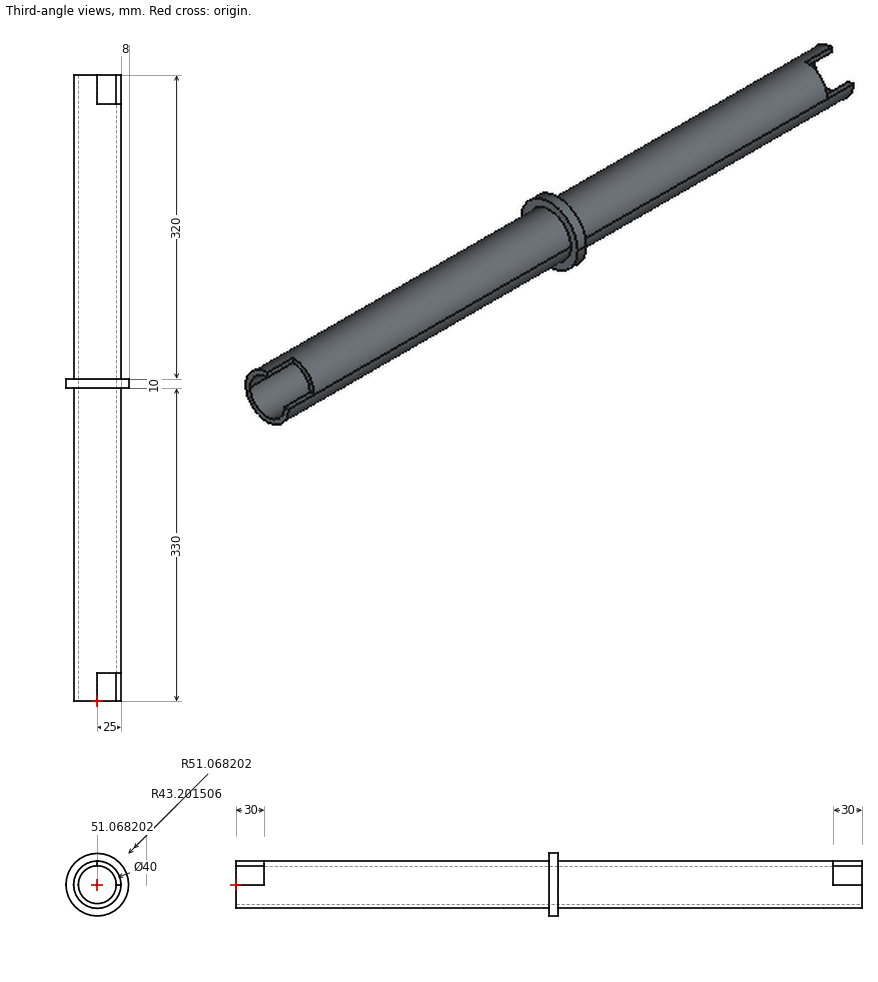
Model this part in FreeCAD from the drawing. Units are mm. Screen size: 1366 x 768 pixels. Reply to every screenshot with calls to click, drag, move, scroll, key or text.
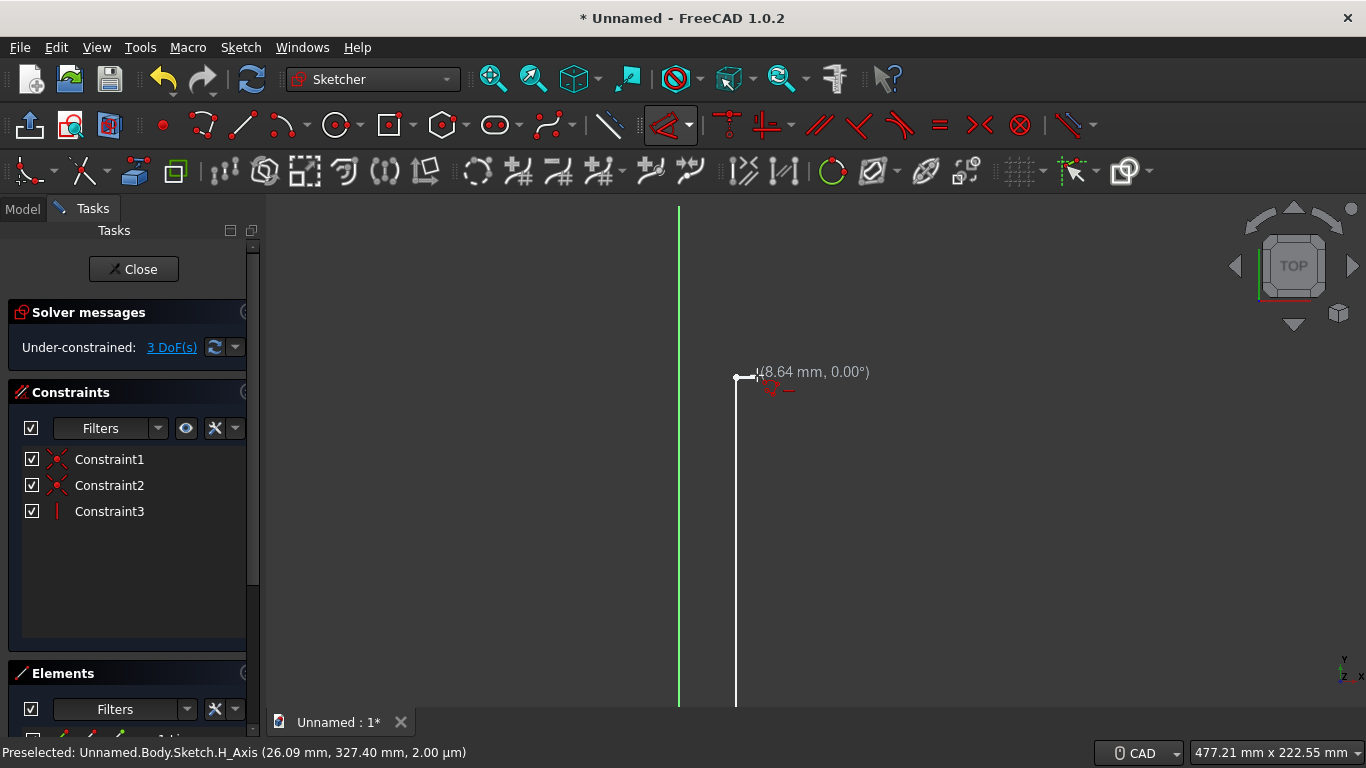
click(755, 374)
click(755, 352)
click(737, 352)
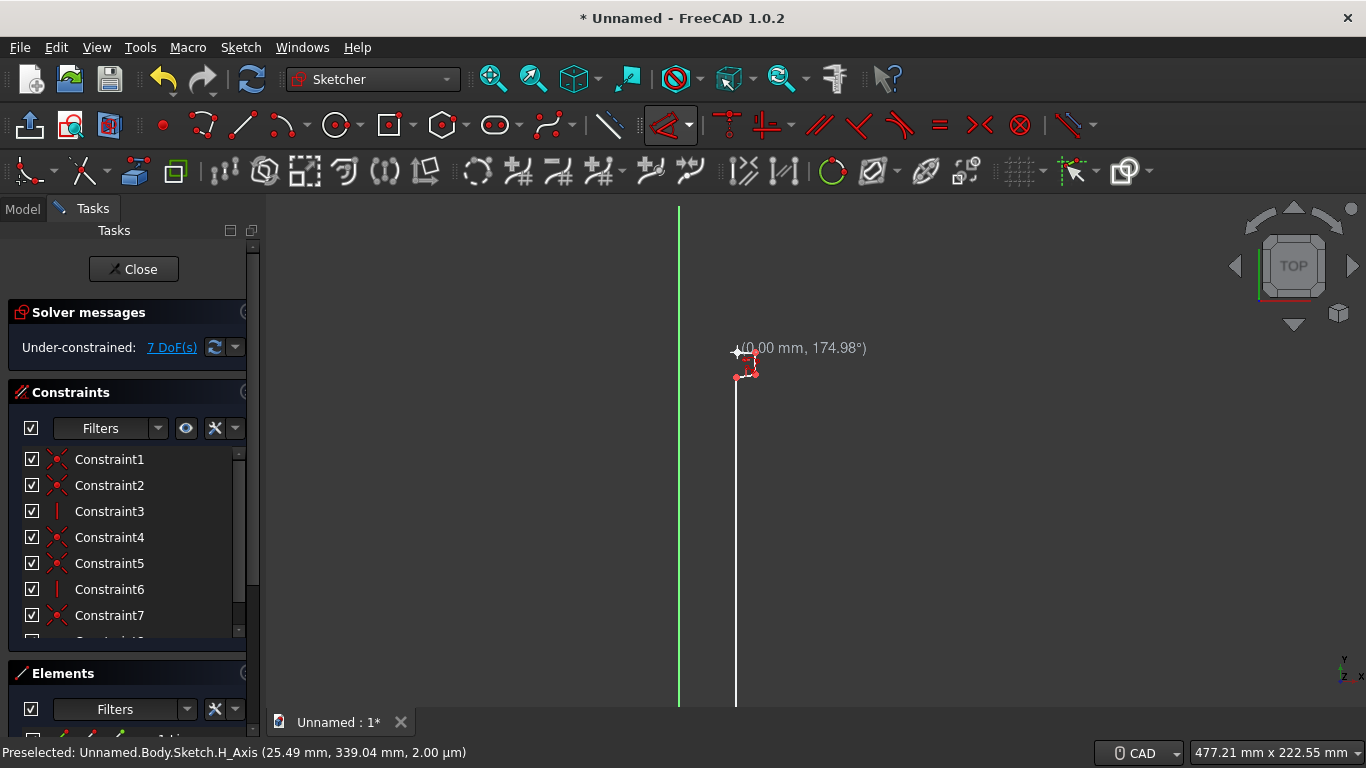
scroll(755, 470, down, 8)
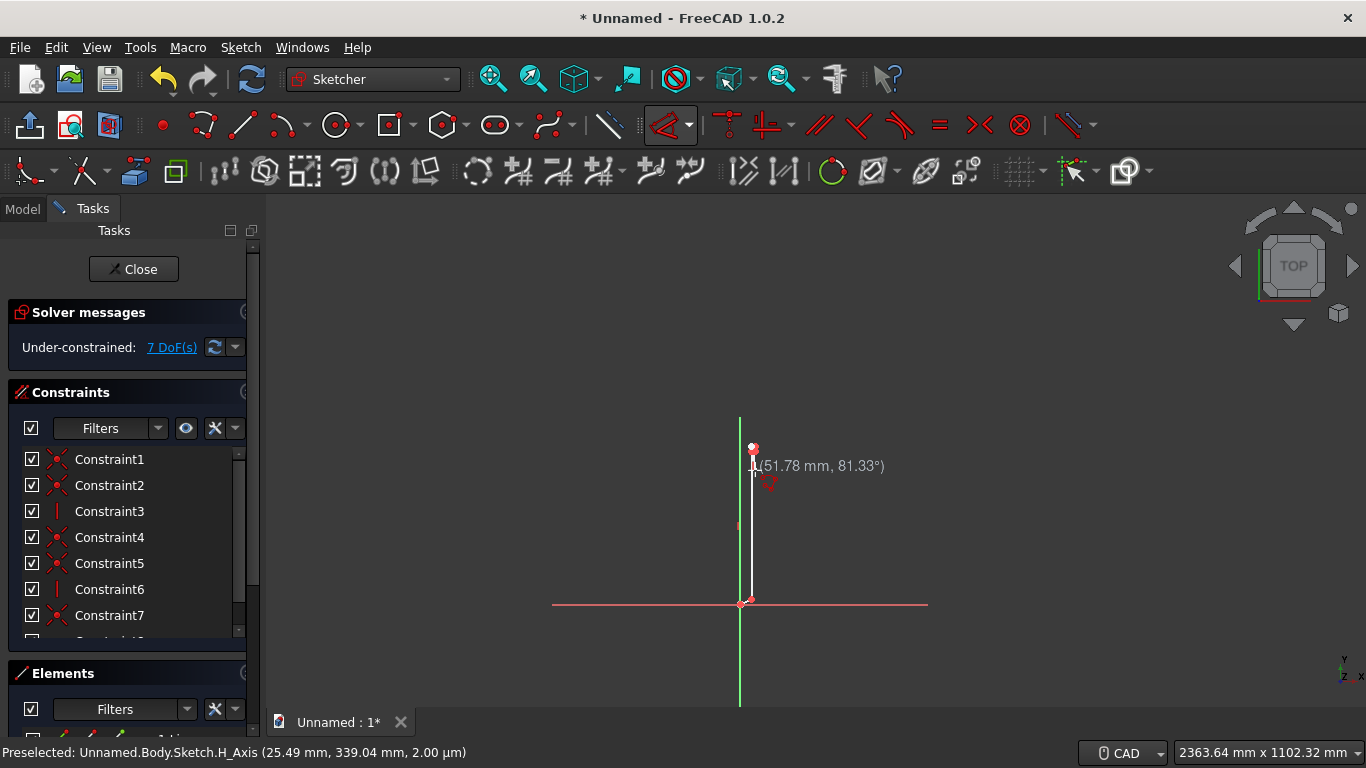
scroll(752, 298, up, 2)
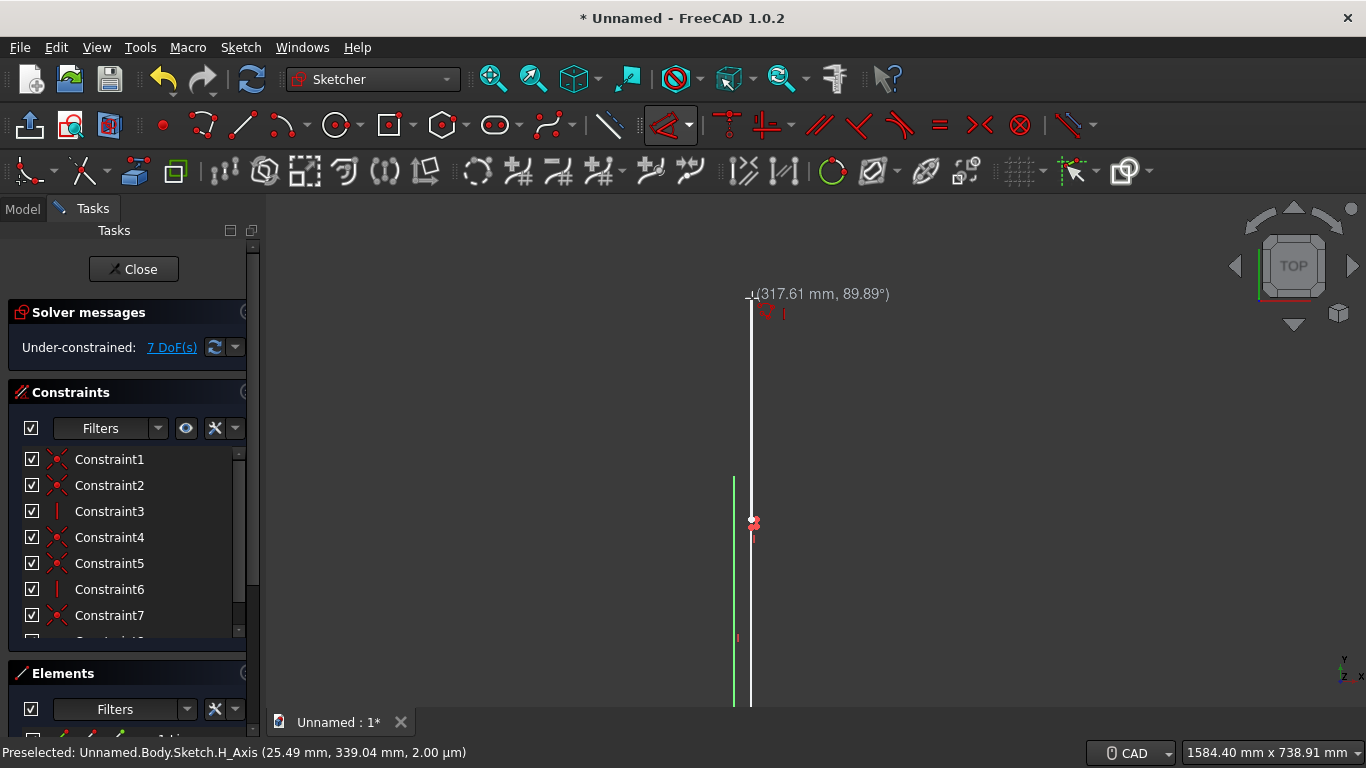
click(751, 297)
click(743, 297)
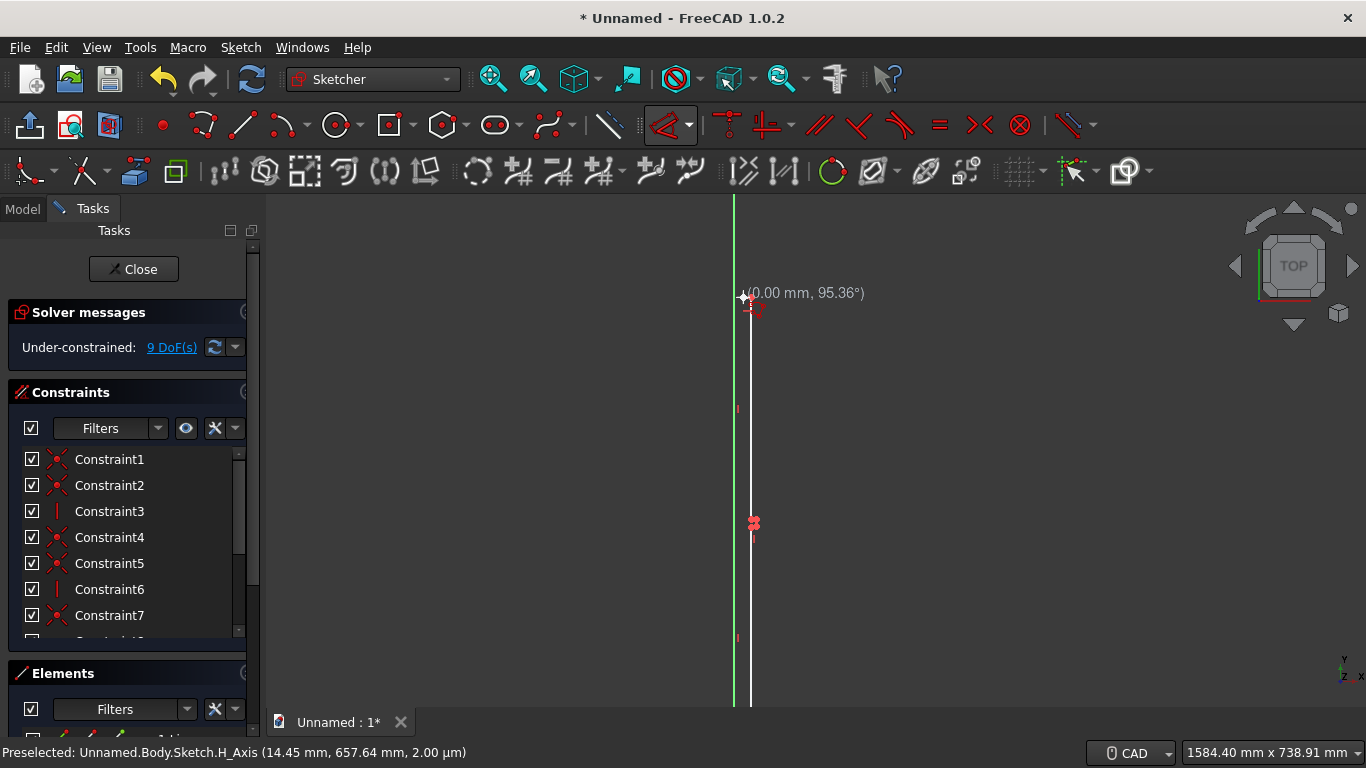
scroll(752, 296, down, 2)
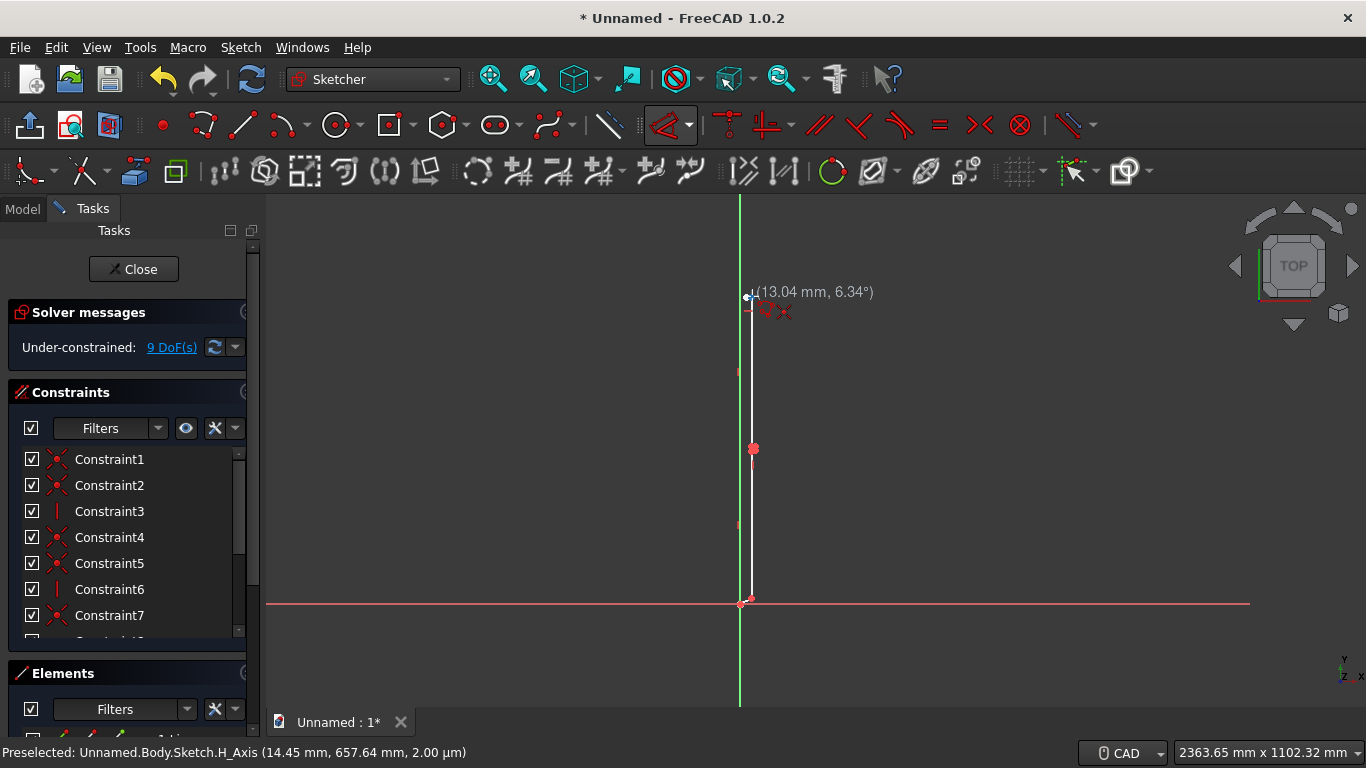
scroll(740, 604, up, 6)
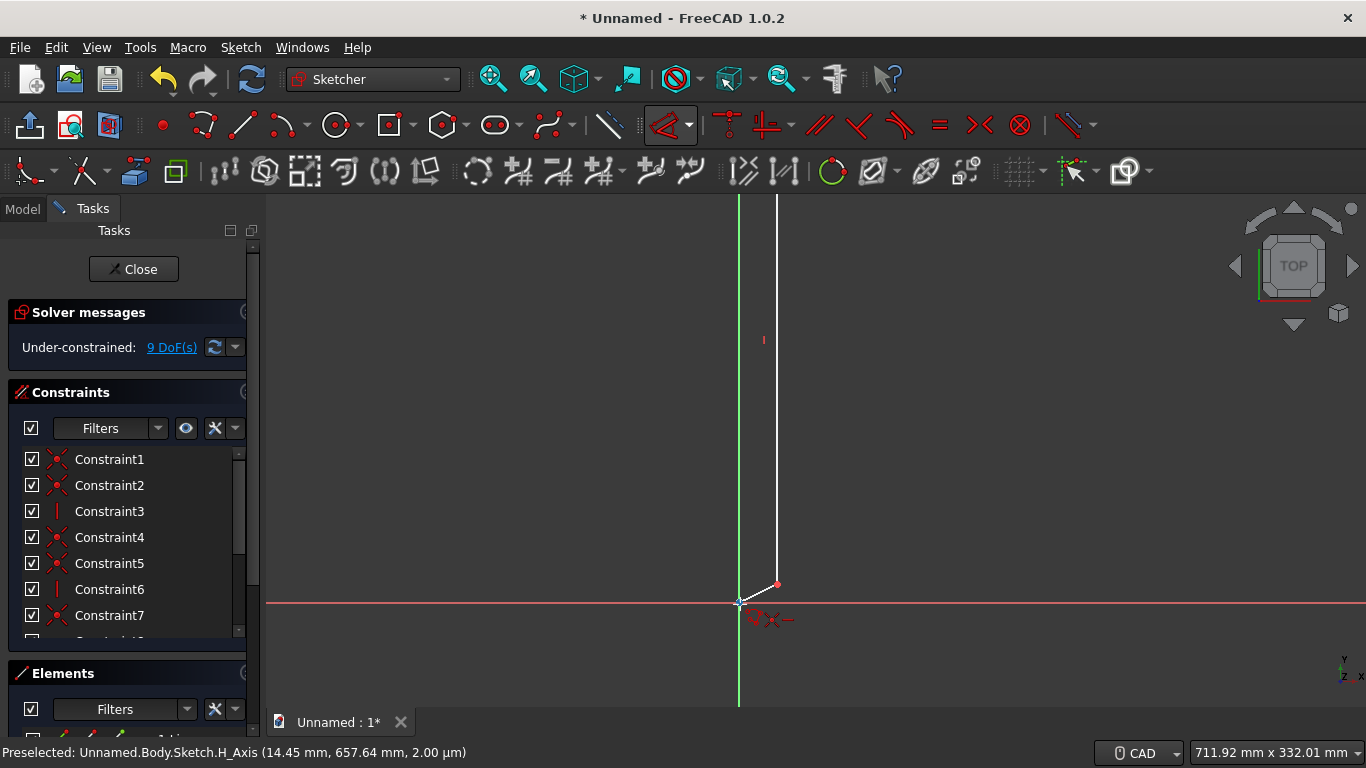
click(739, 603)
key(Escape)
key(Escape)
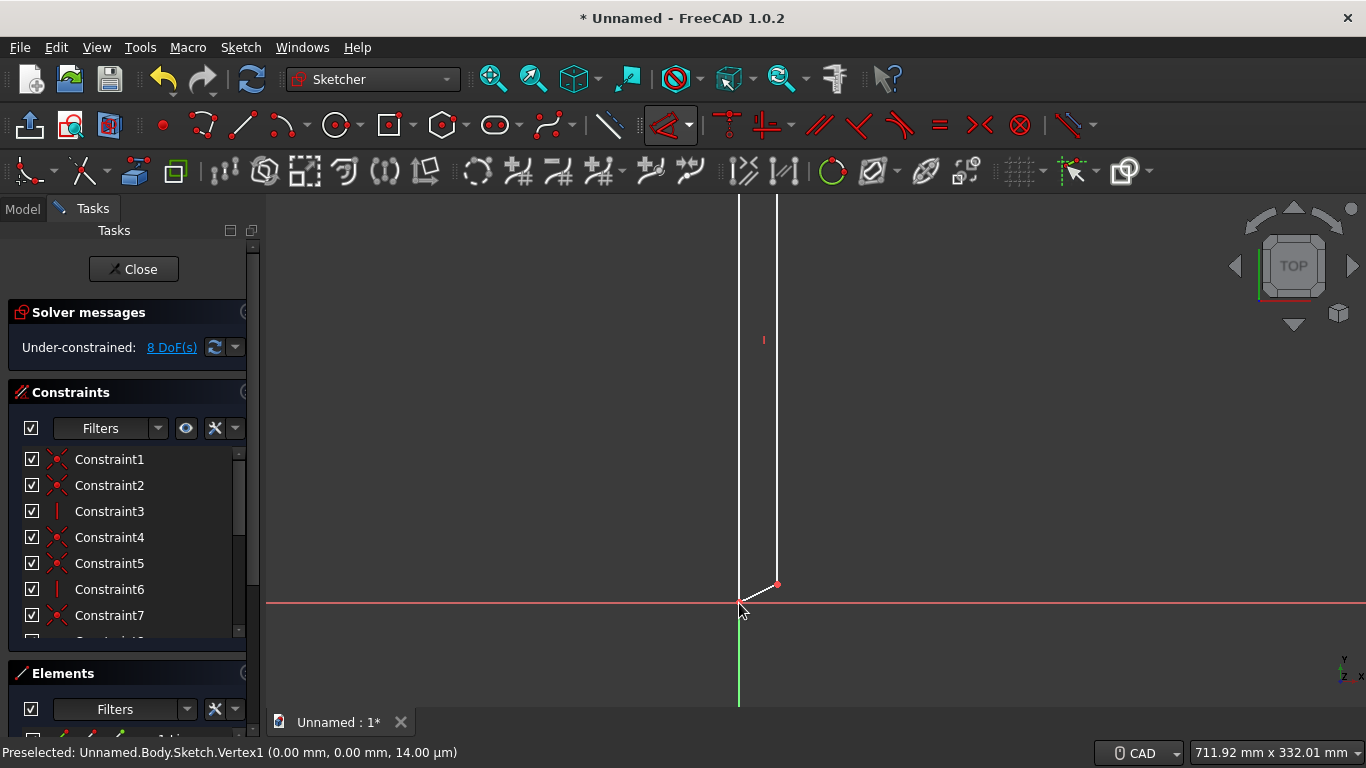
click(766, 590)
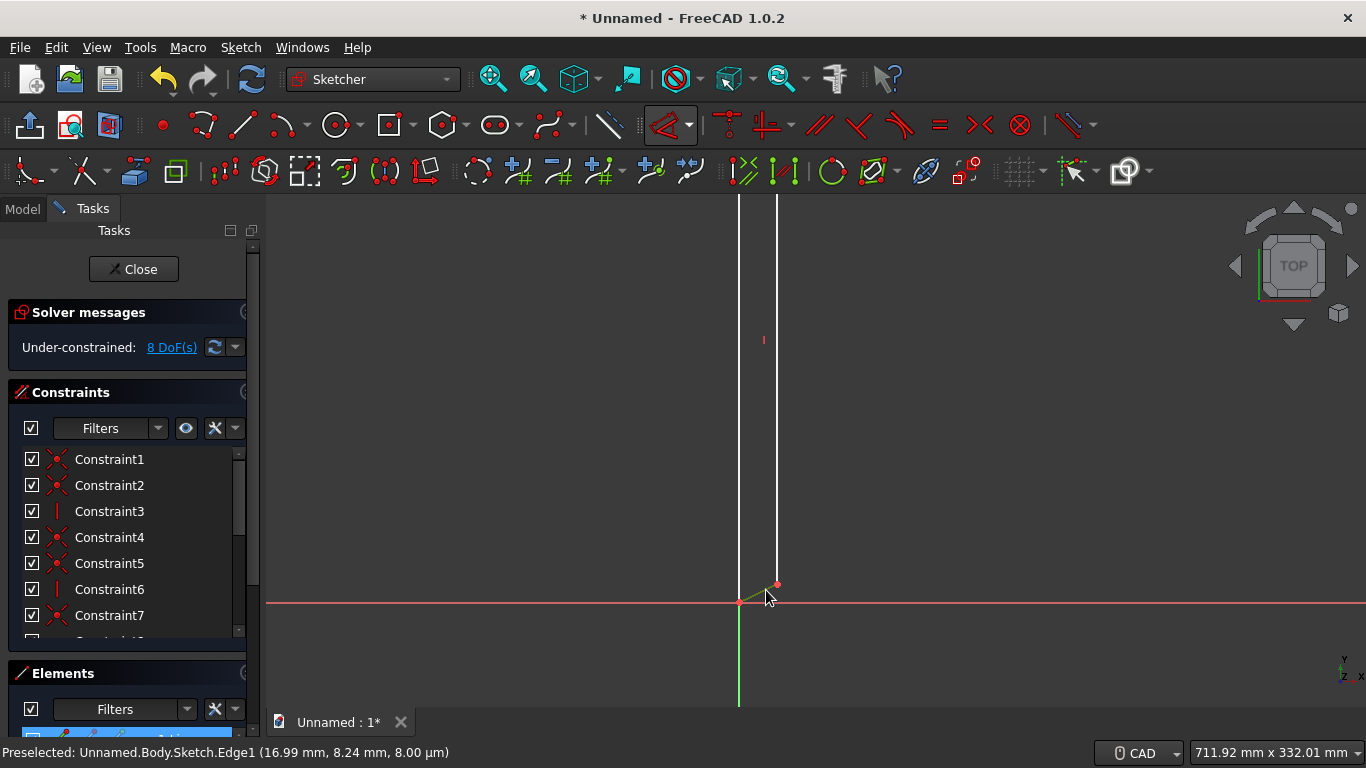
click(794, 126)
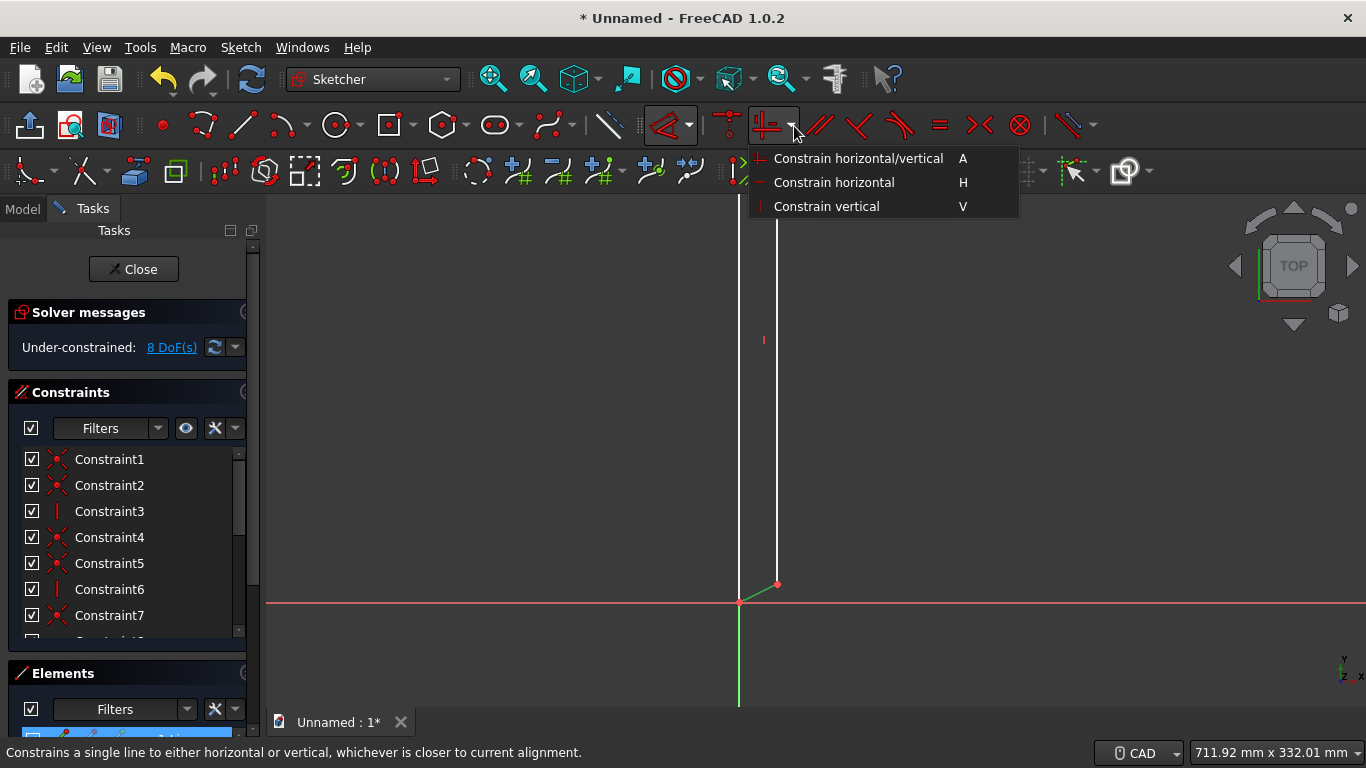
click(884, 182)